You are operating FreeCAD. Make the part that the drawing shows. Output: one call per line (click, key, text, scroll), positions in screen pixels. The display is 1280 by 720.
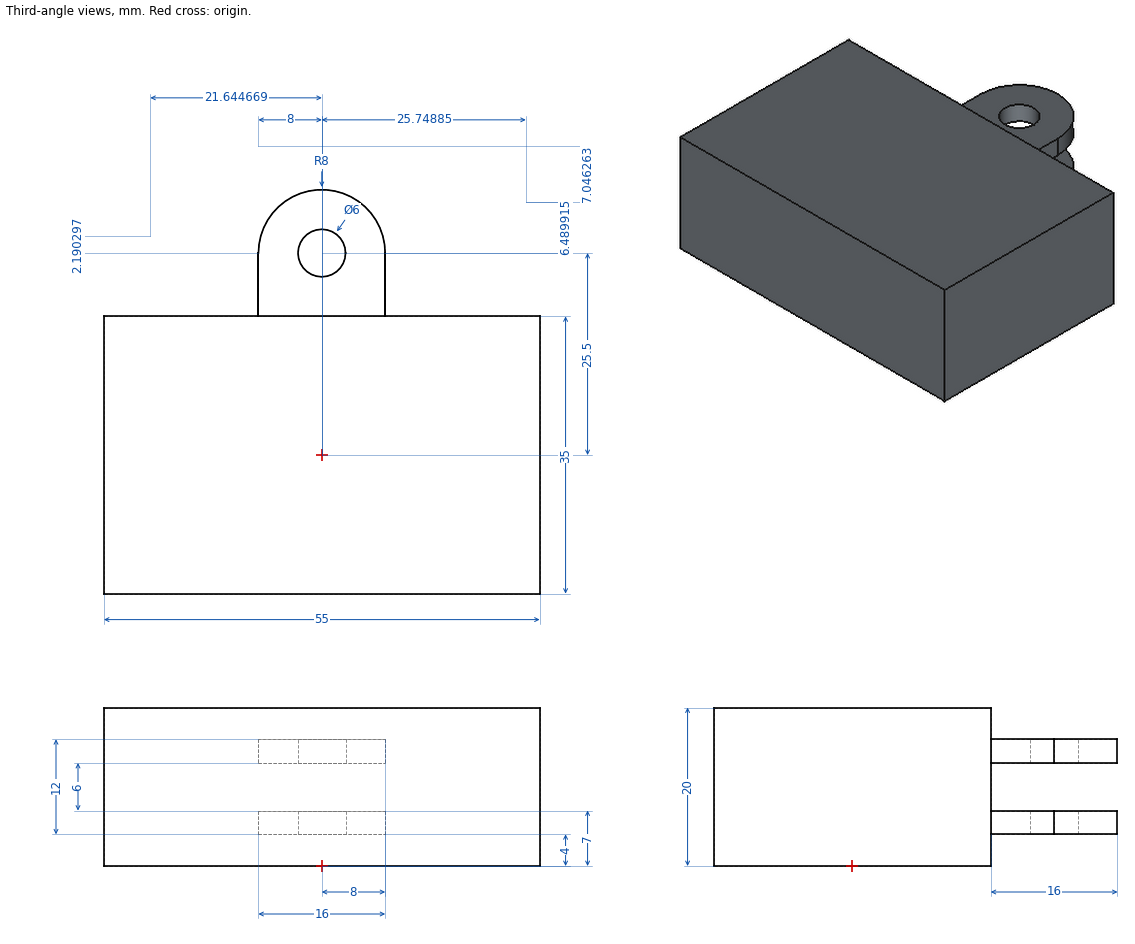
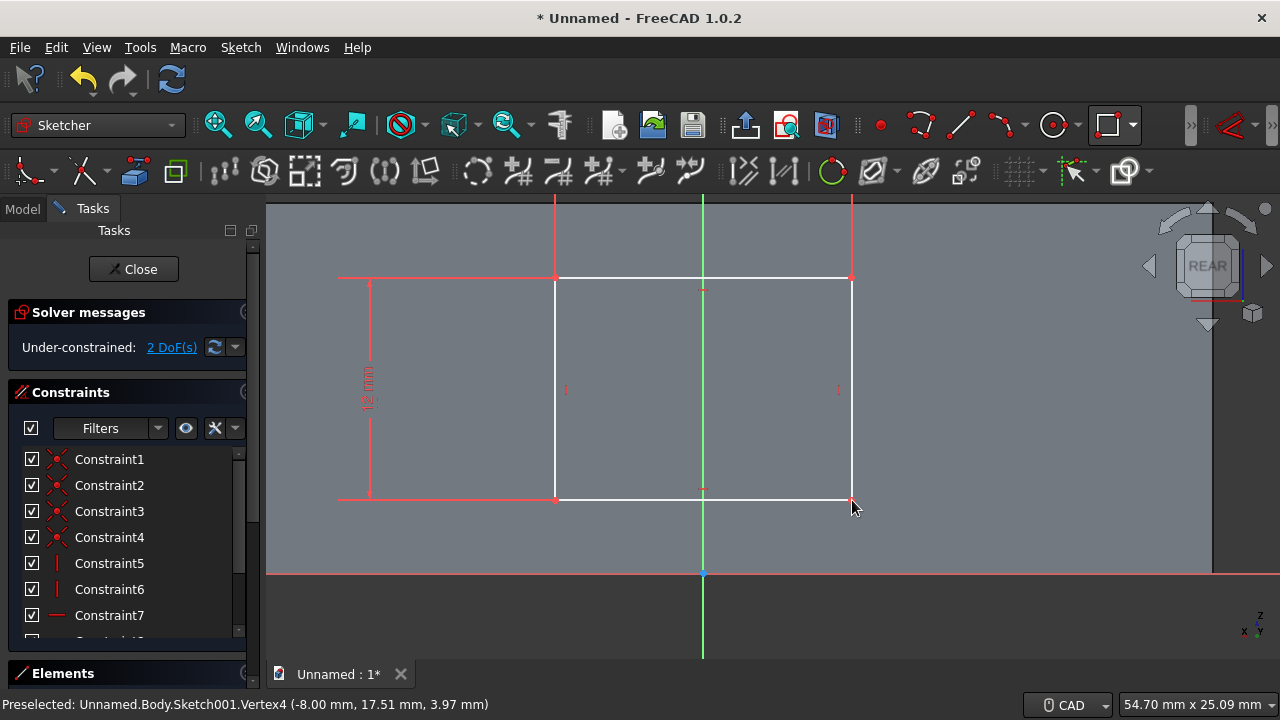
click(555, 278)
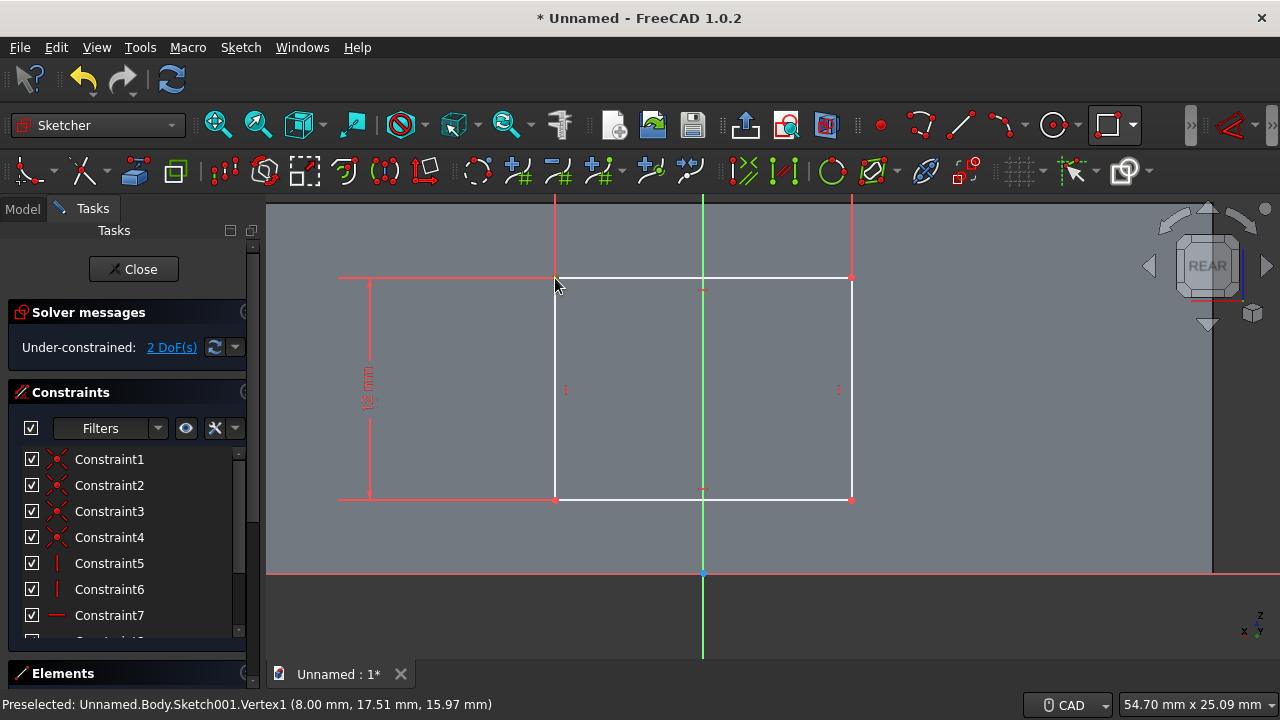
key(l)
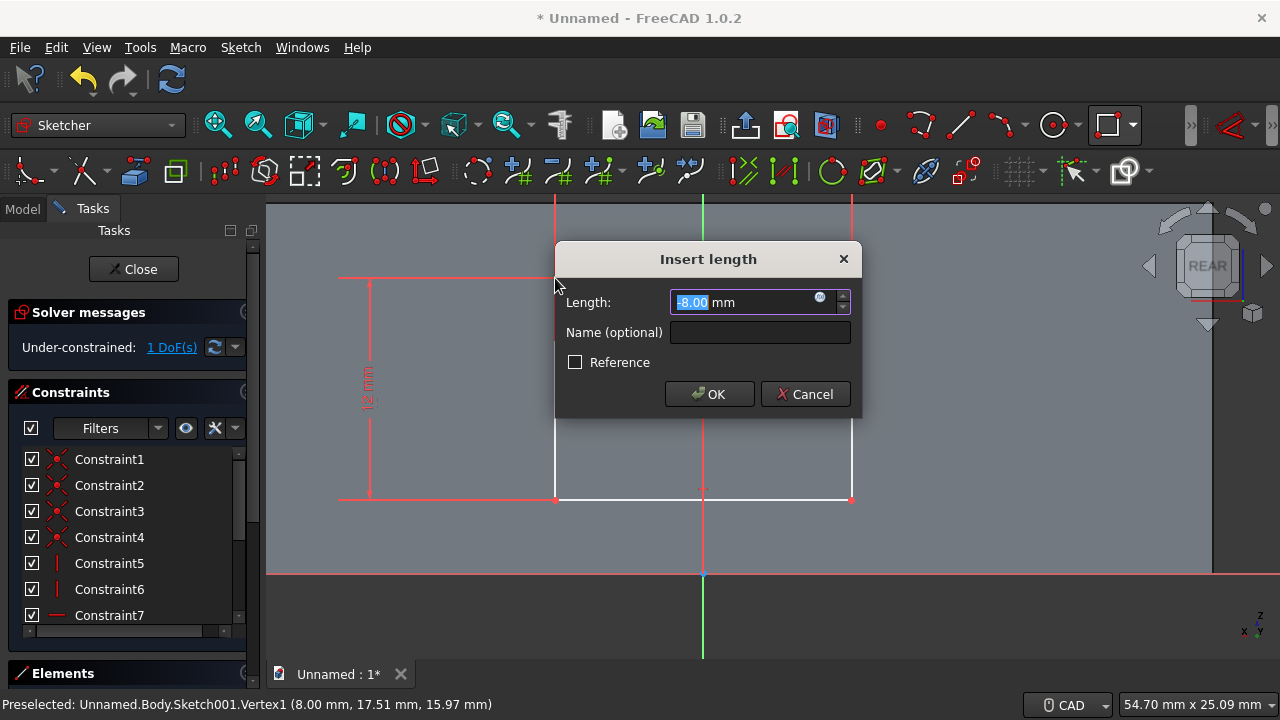
text(-8)
key(Return)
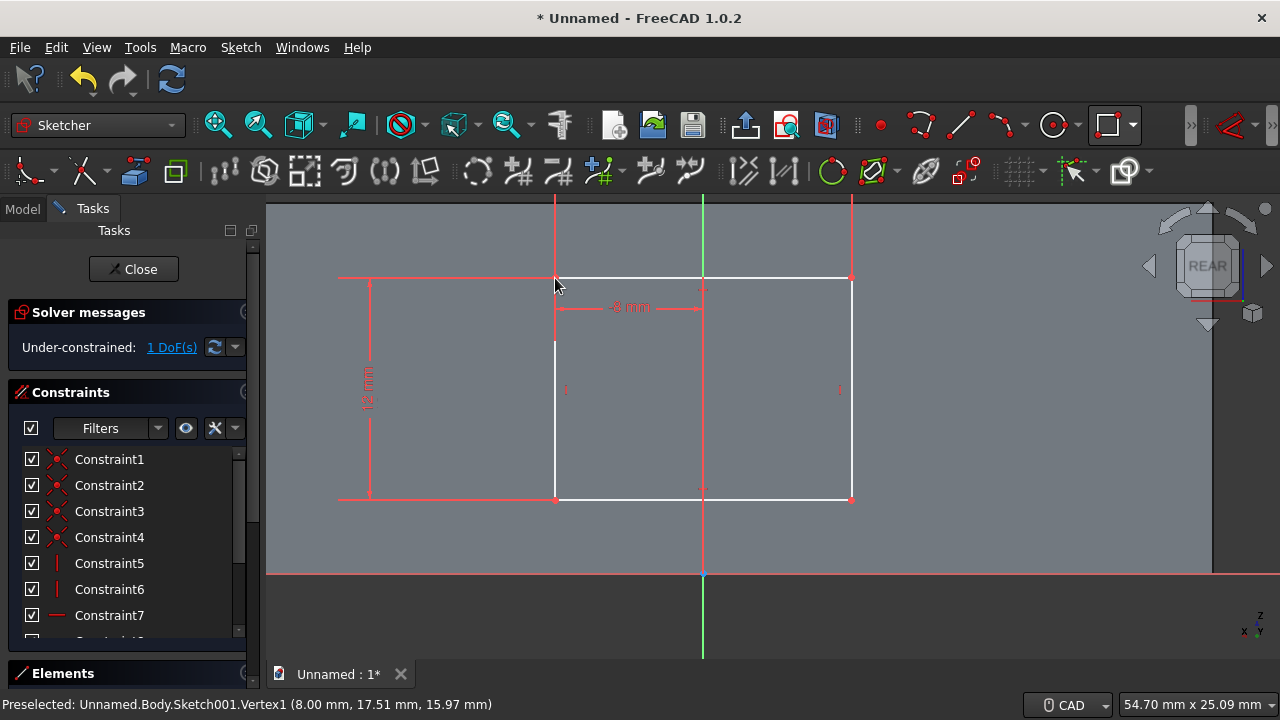
click(555, 500)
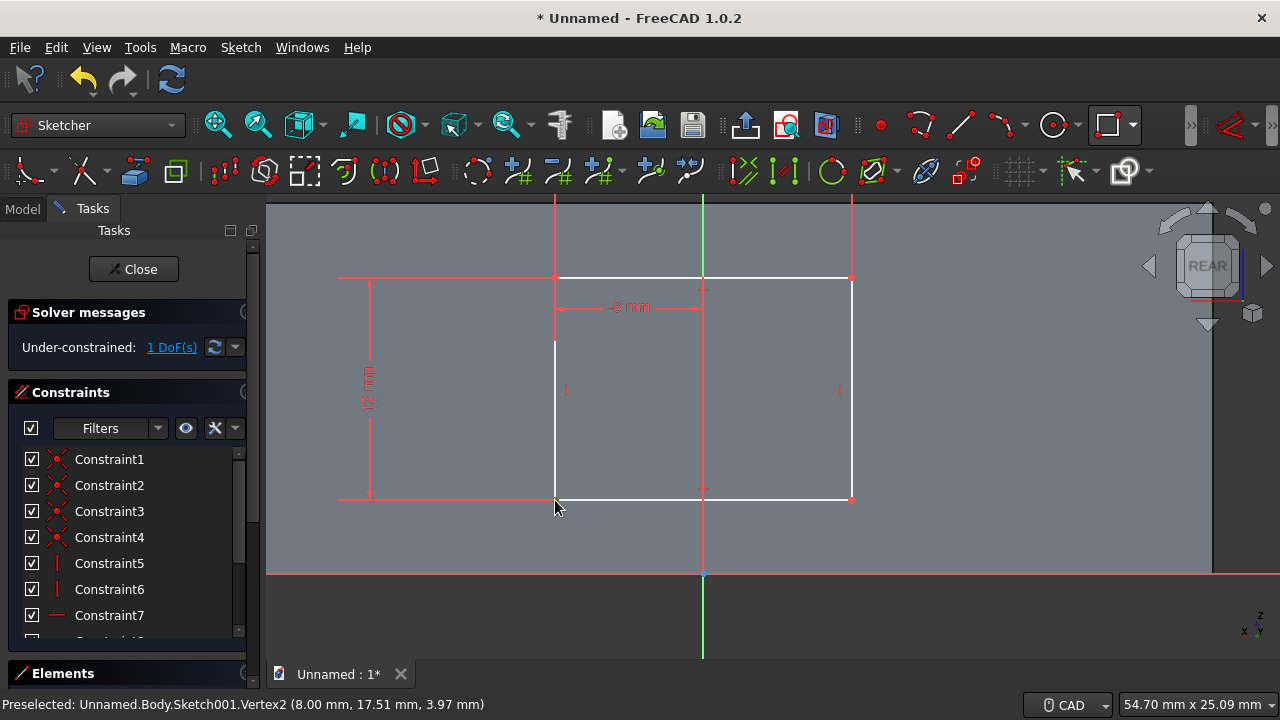
click(1258, 126)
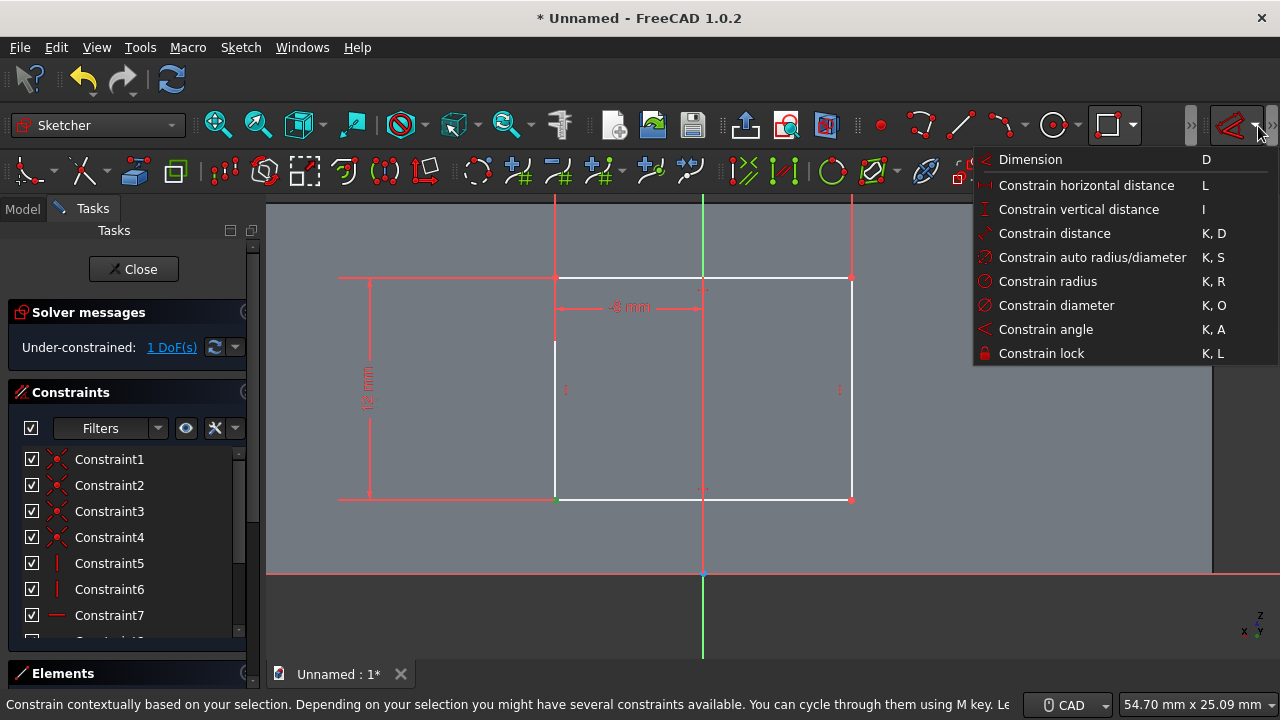
click(1126, 209)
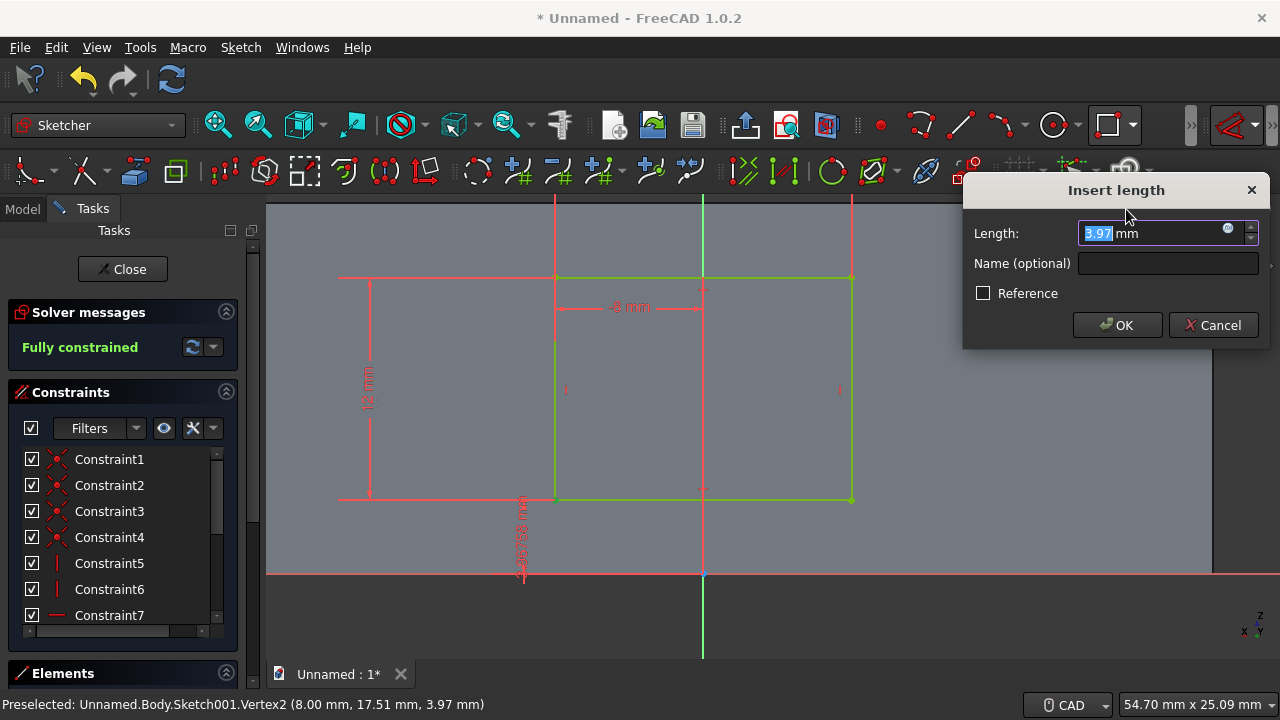
text(4)
key(Return)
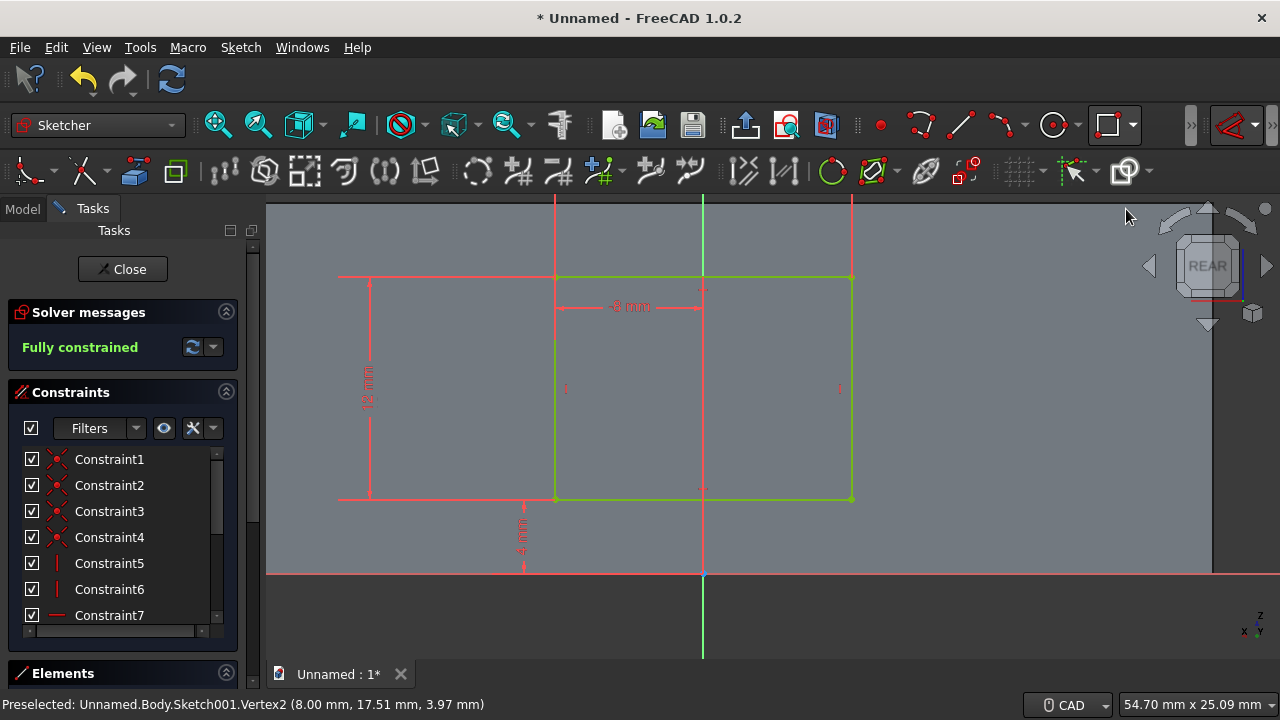
click(123, 269)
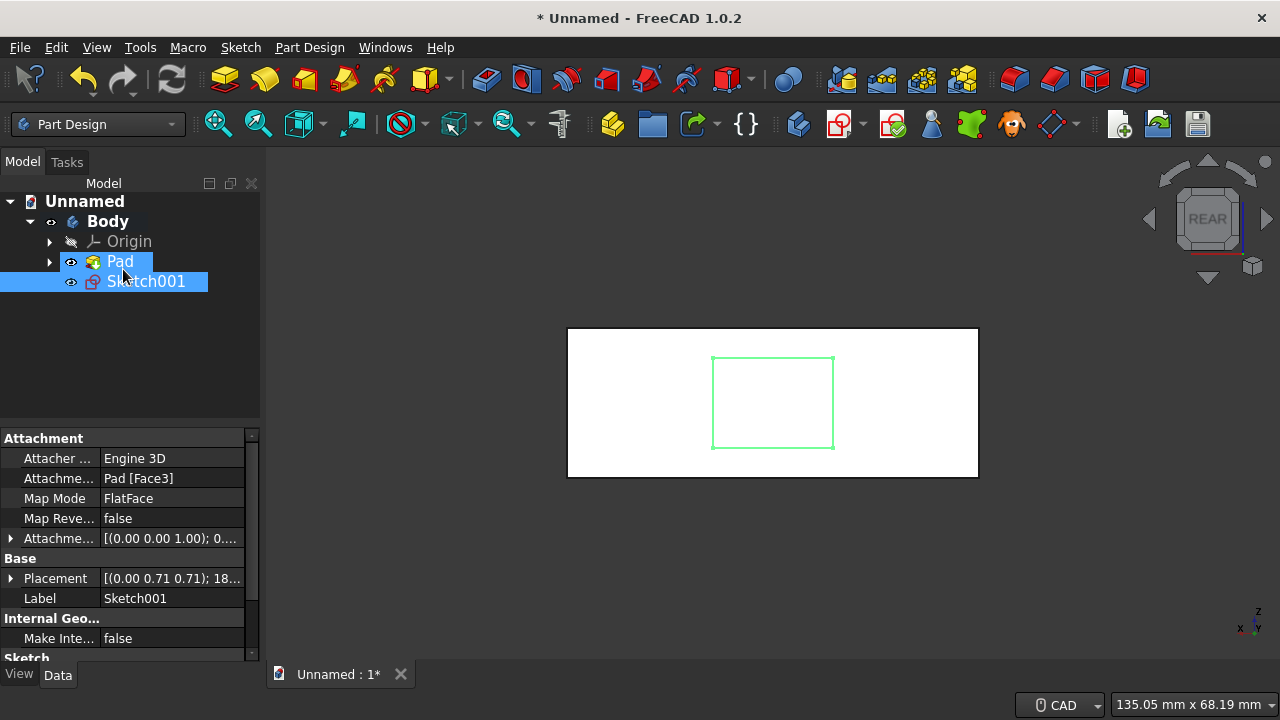
click(226, 80)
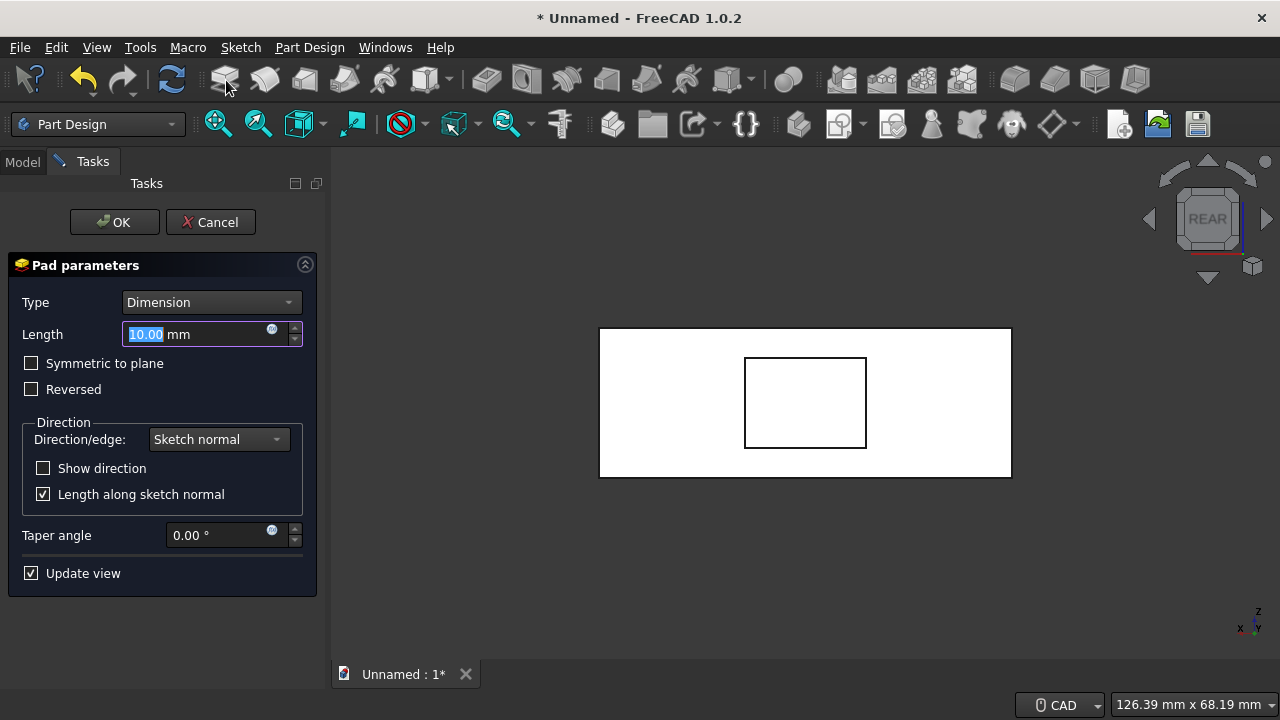
text(16)
key(Tab)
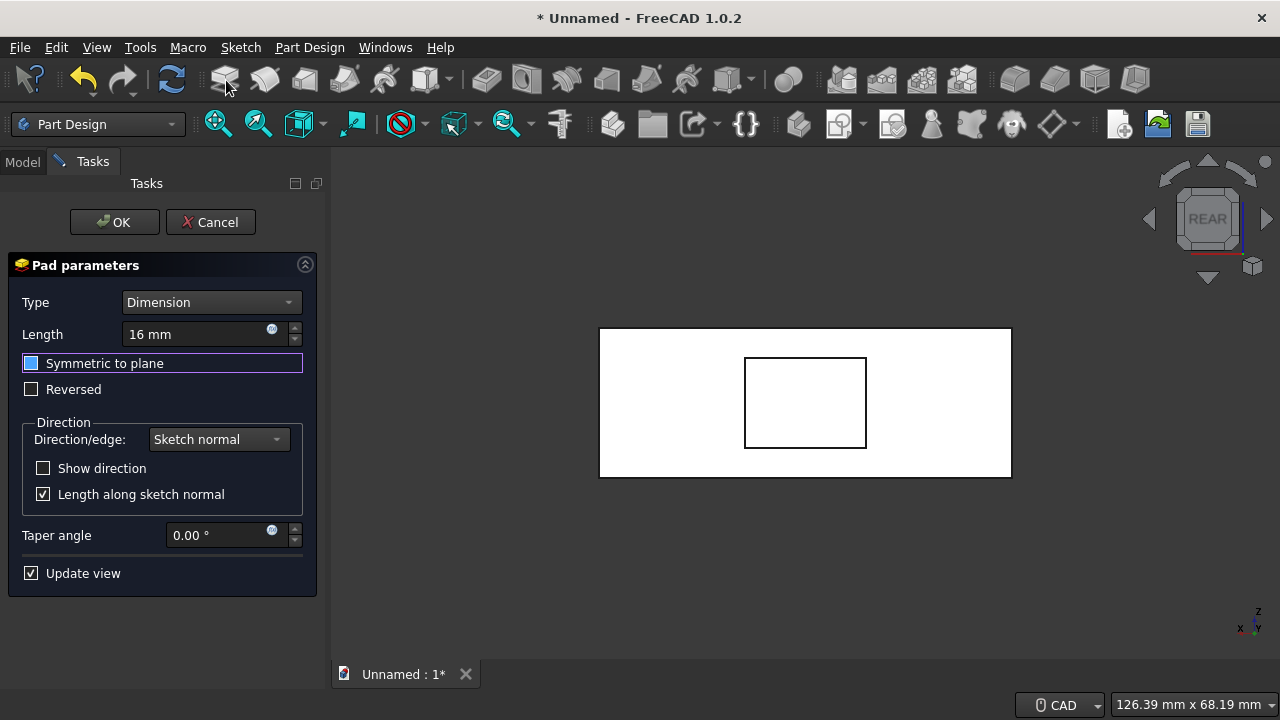
click(115, 222)